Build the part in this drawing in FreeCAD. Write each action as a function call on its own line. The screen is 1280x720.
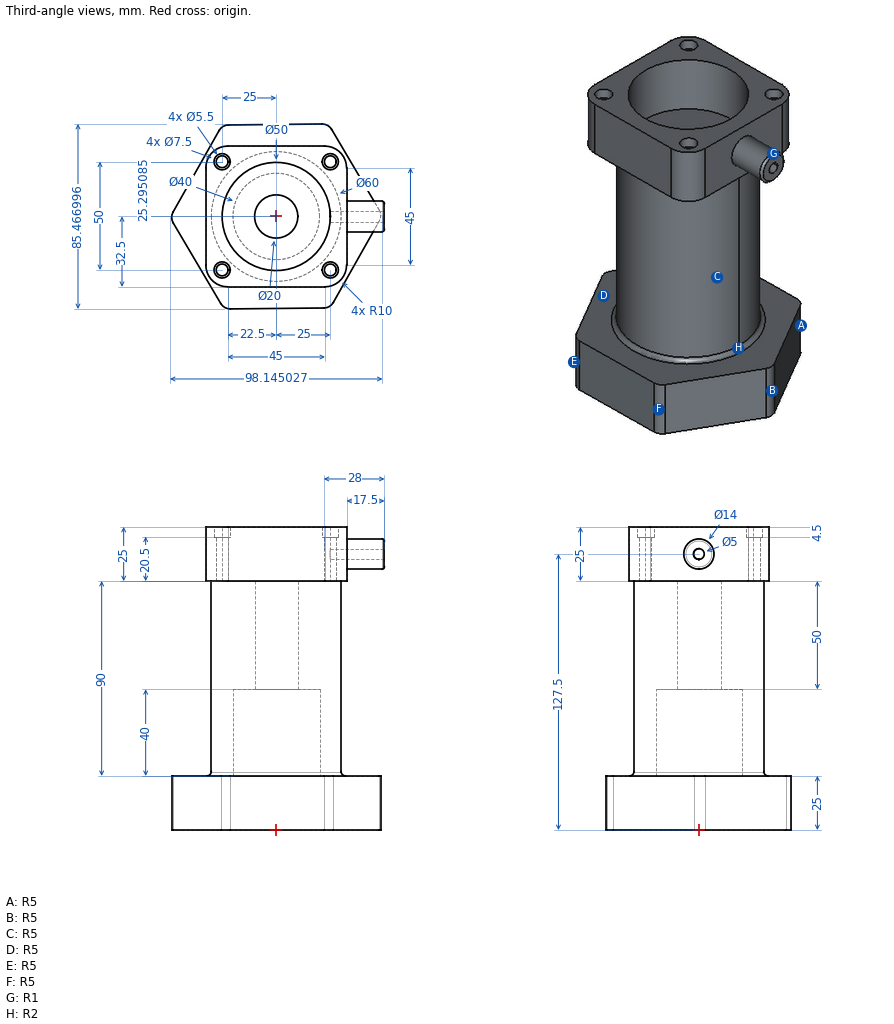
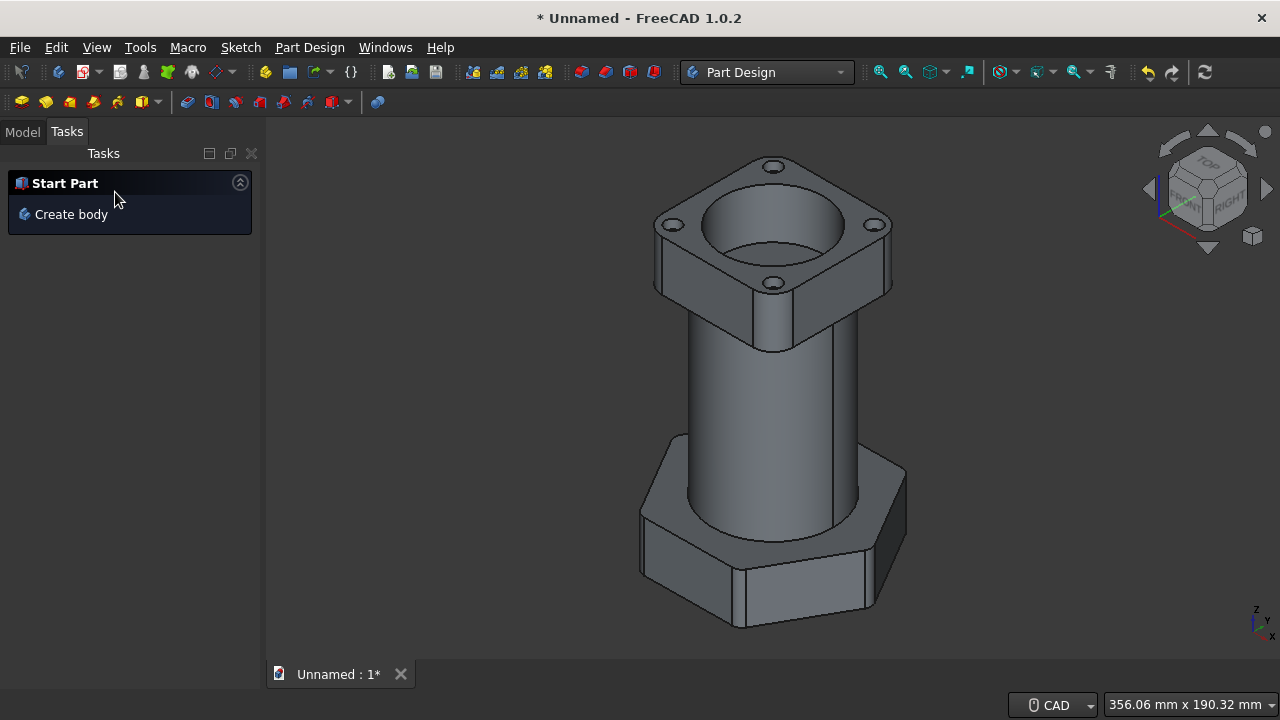
key(2)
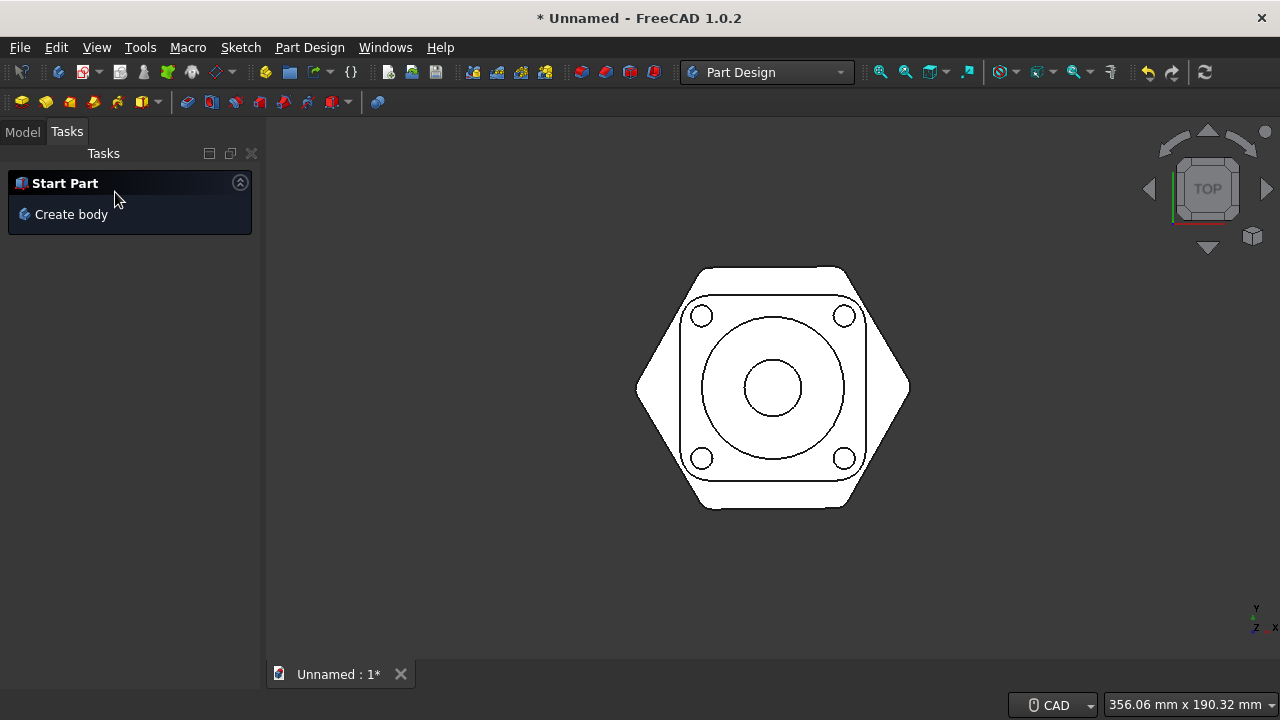
click(844, 315)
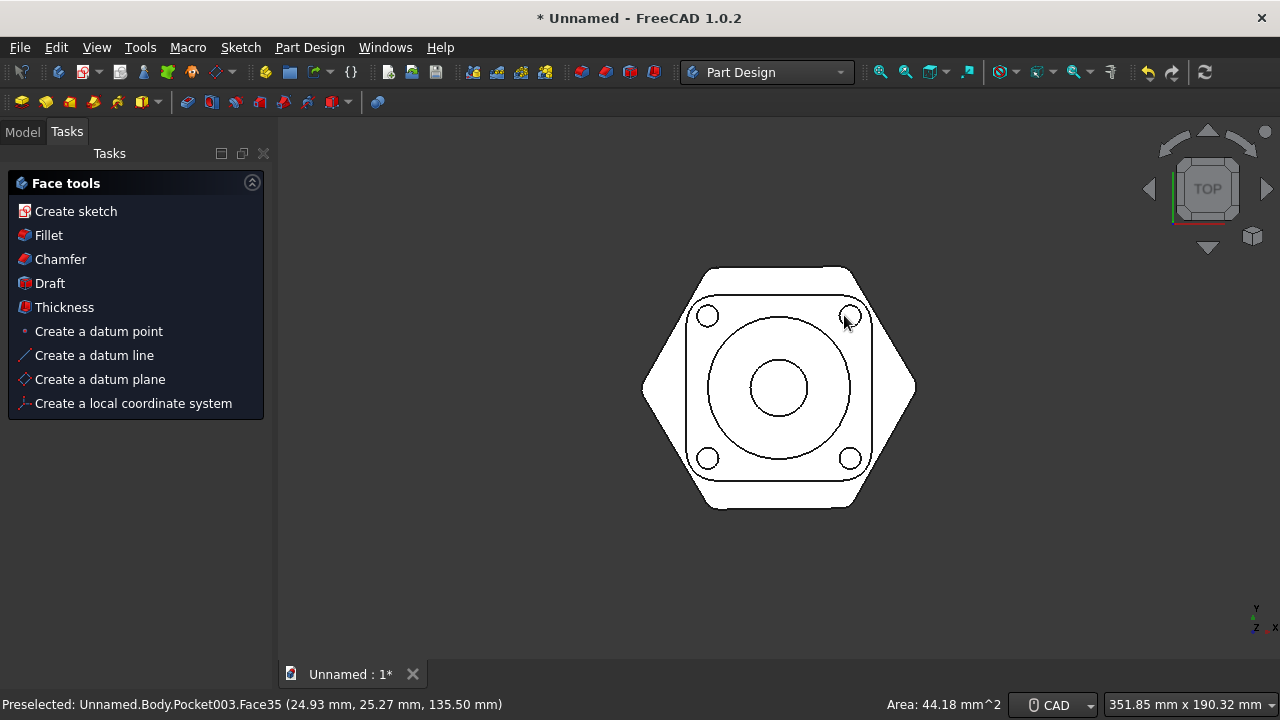
click(84, 72)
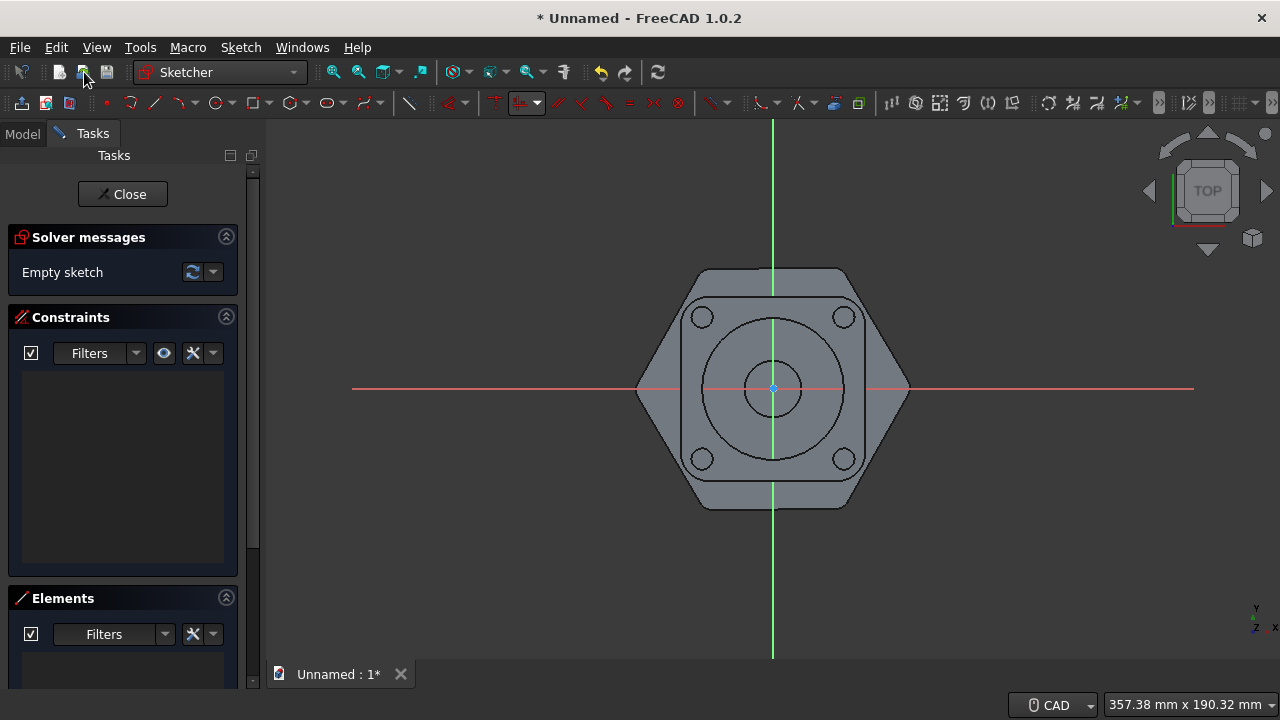
scroll(829, 387, up, 4)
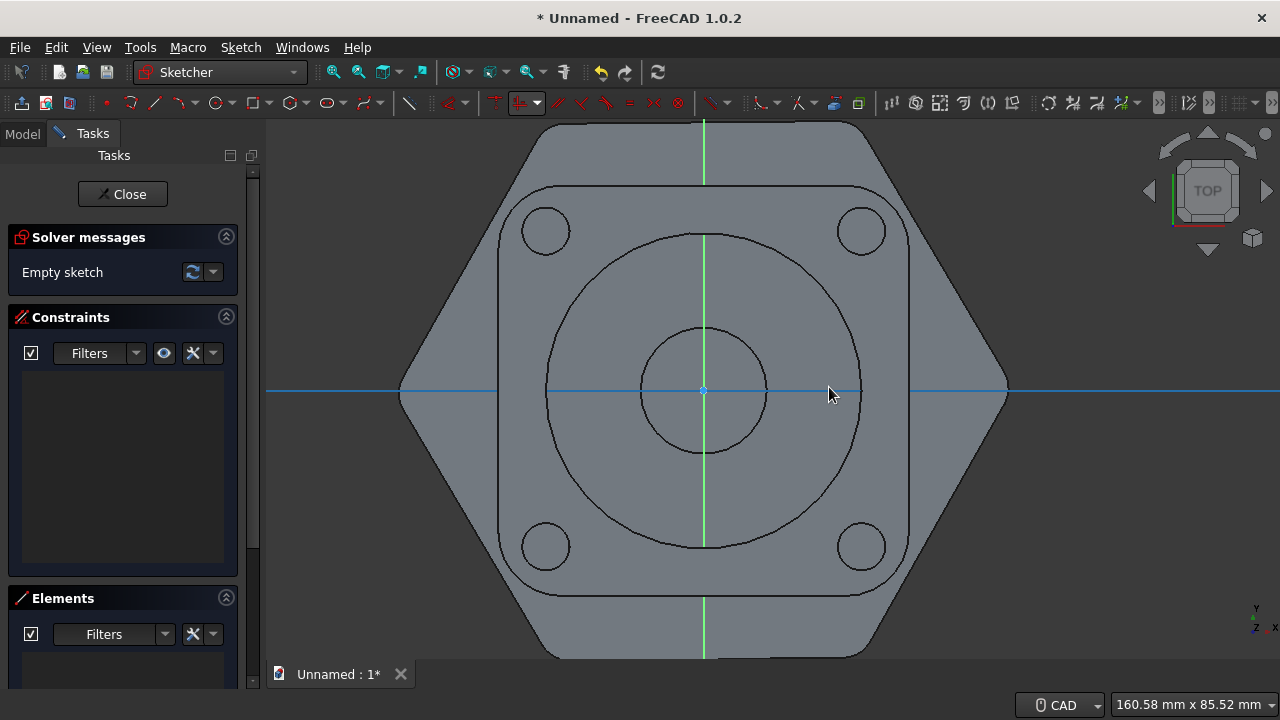
click(216, 104)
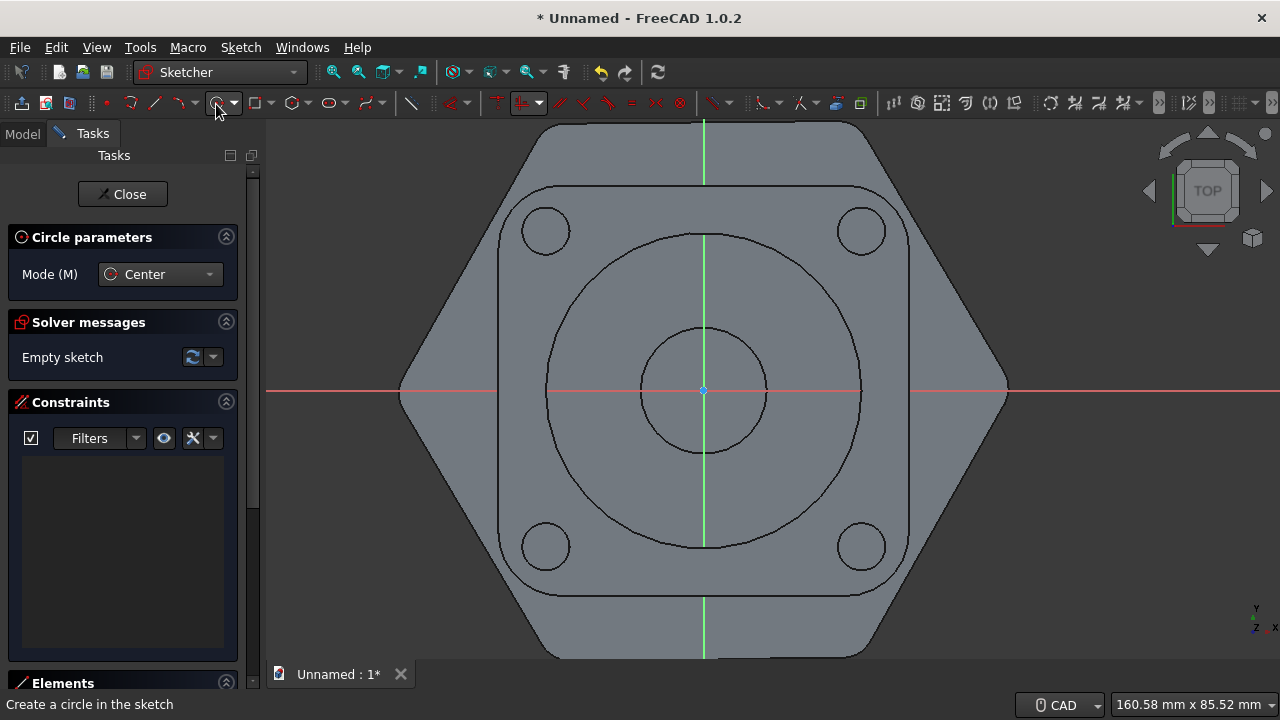
scroll(546, 231, up, 2)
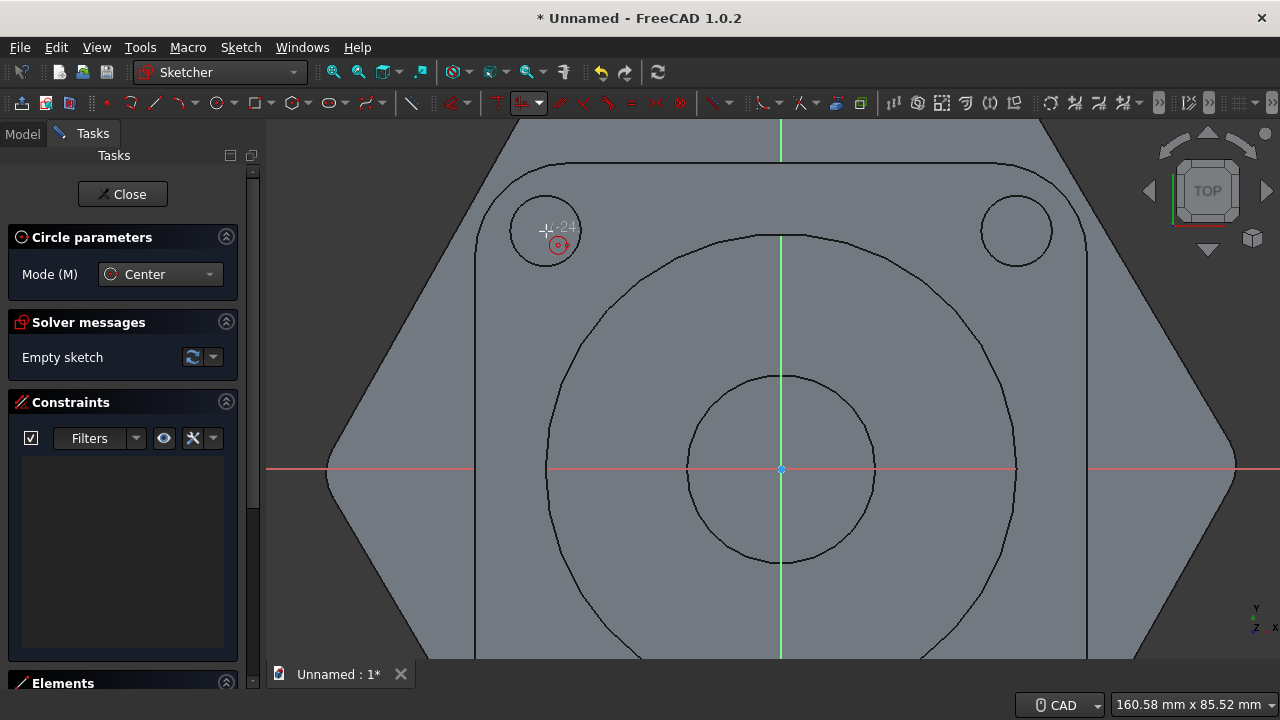
click(546, 231)
click(564, 213)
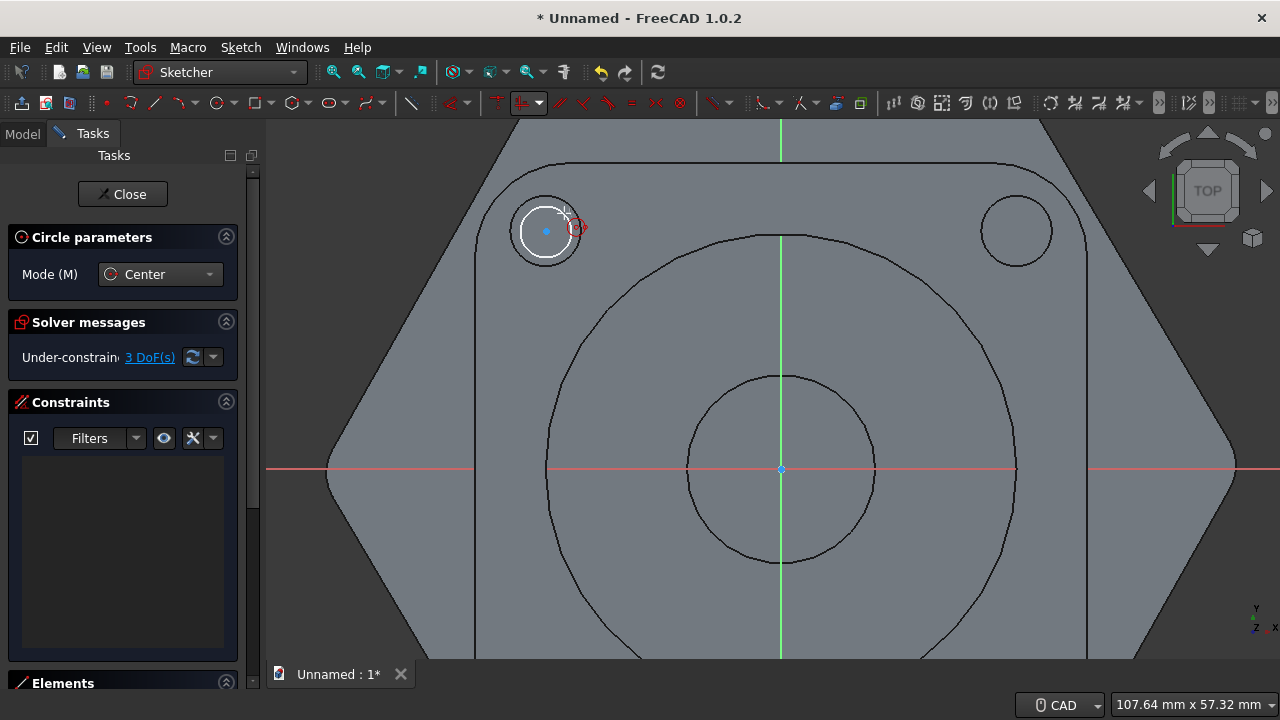
click(1017, 231)
click(1035, 213)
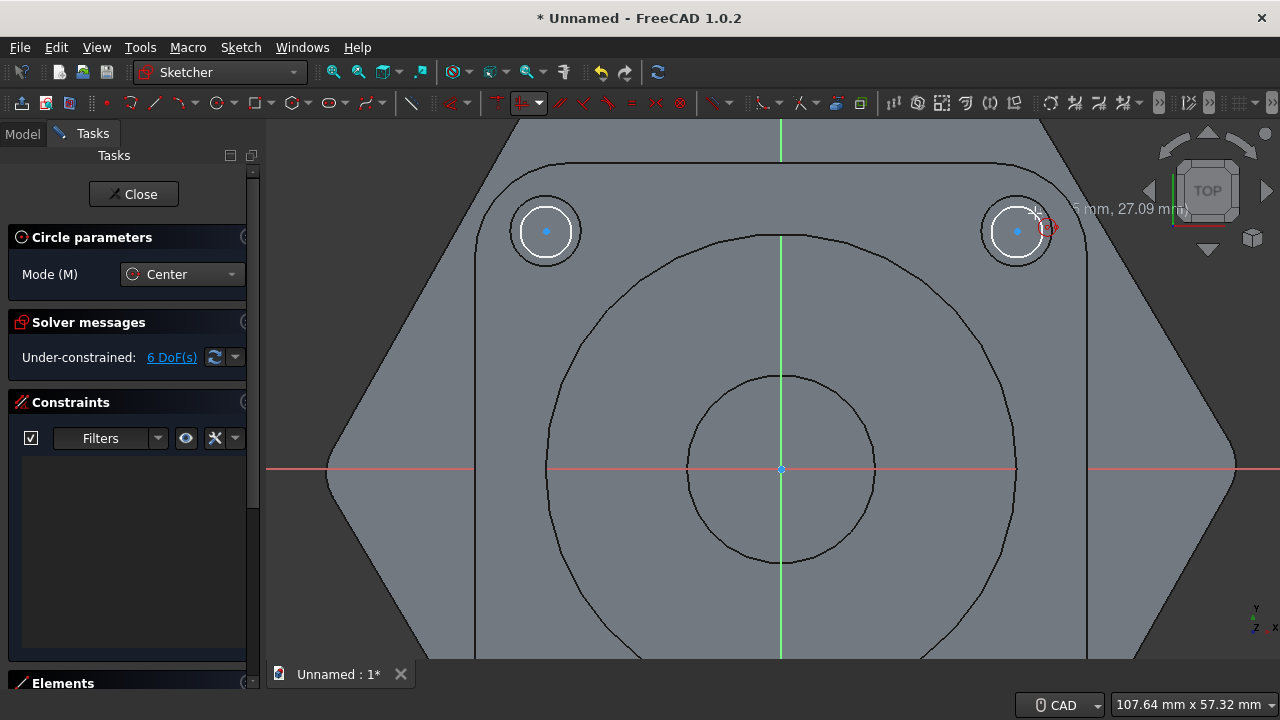
scroll(549, 232, down, 2)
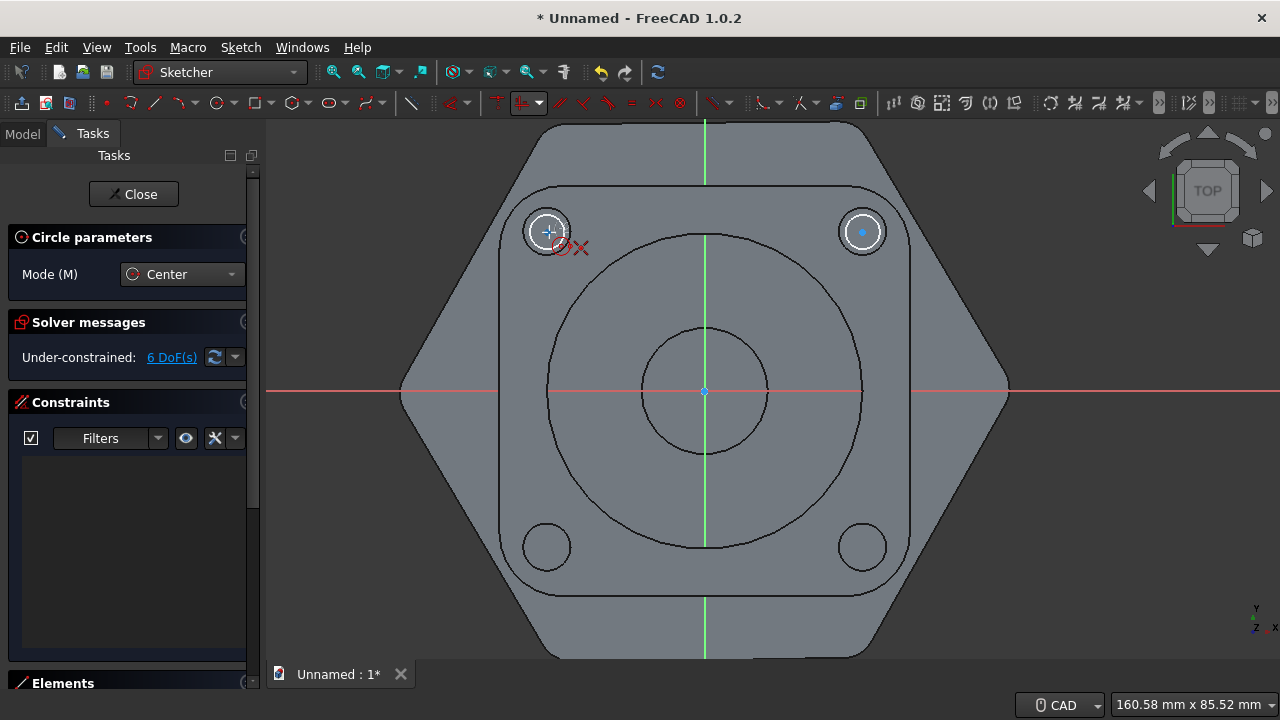
scroll(863, 547, up, 2)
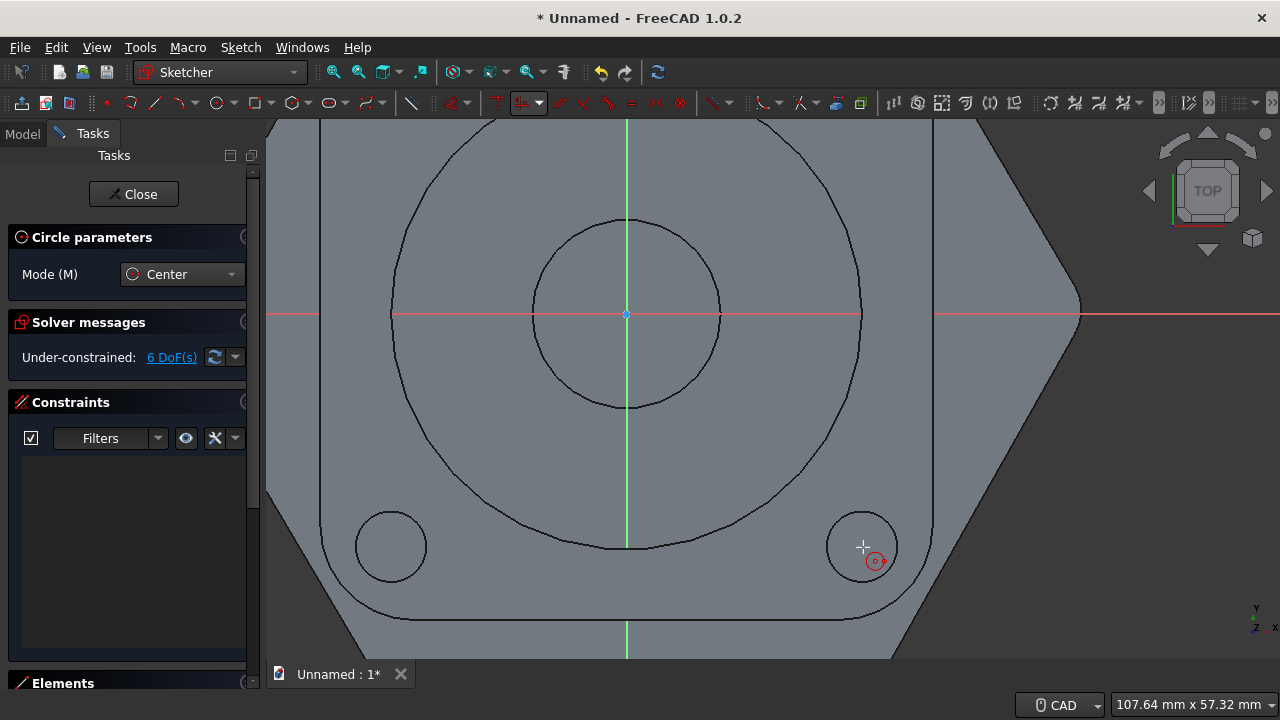
click(862, 547)
click(880, 528)